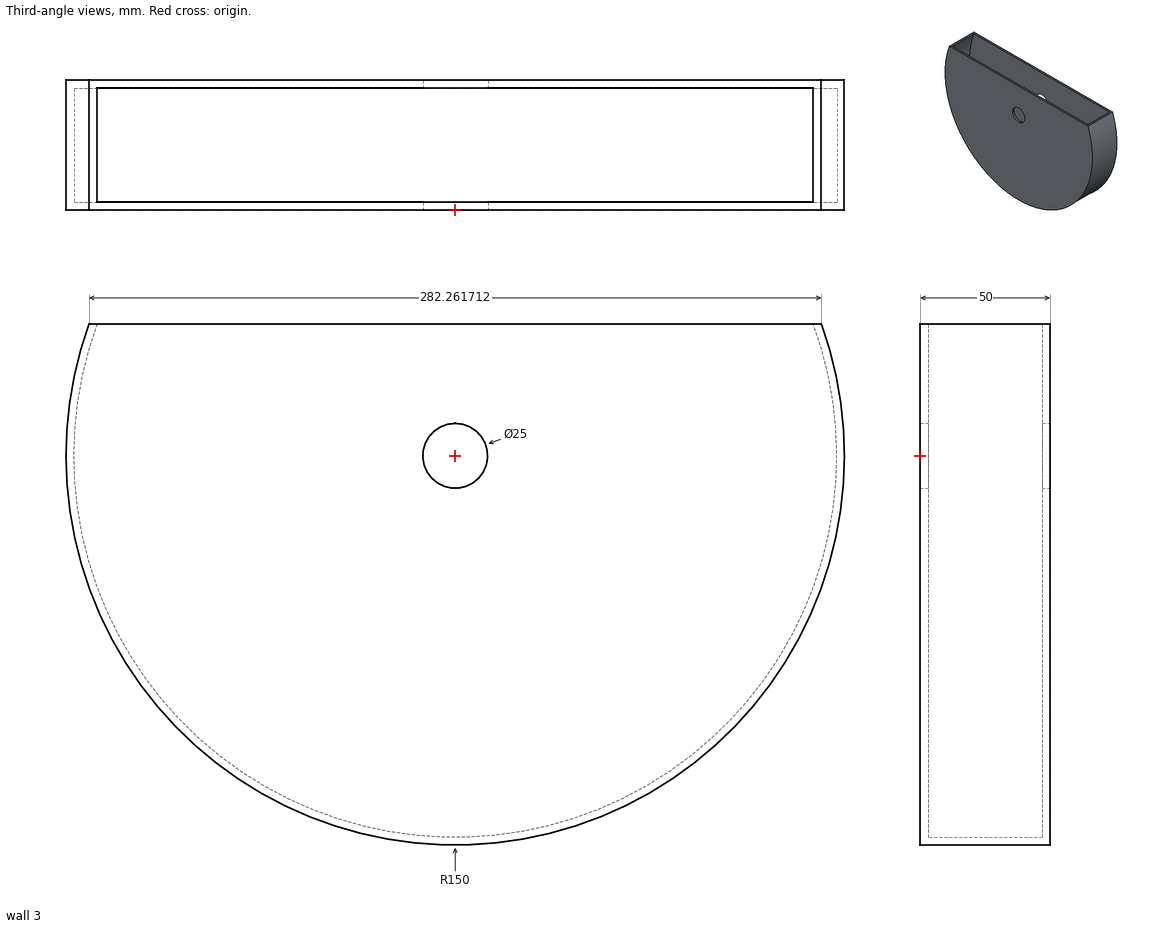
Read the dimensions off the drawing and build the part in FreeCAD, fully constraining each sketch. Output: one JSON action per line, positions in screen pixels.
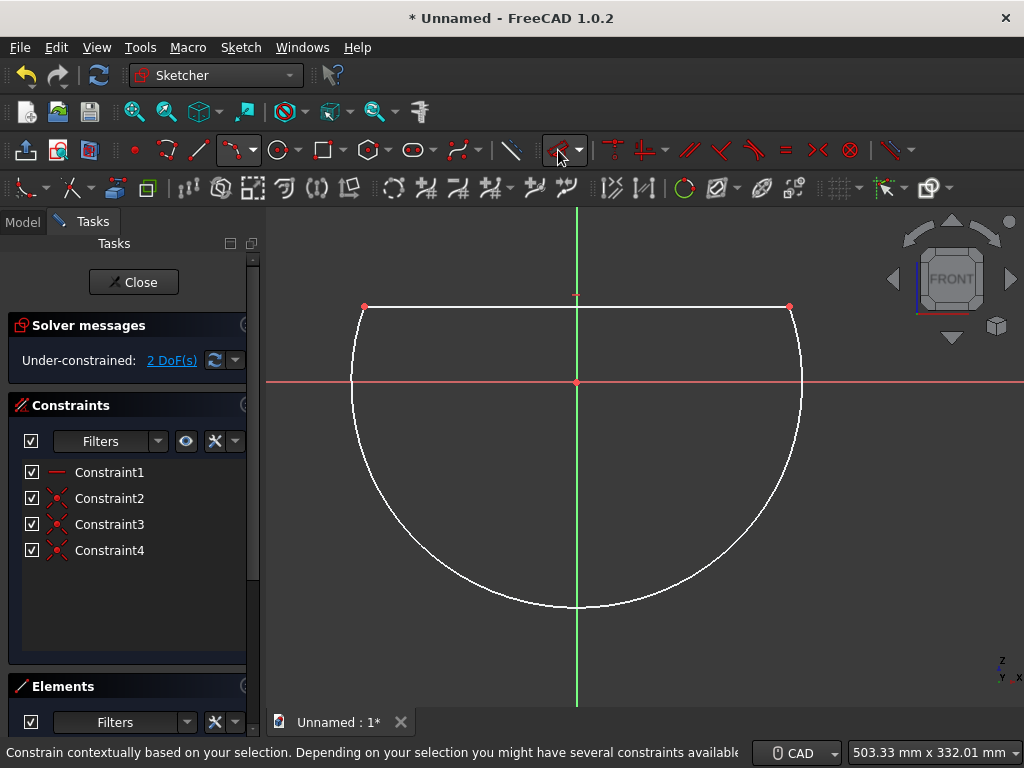
{"action": "left_click", "coordinate": [421, 545]}
{"action": "left_click", "coordinate": [399, 568]}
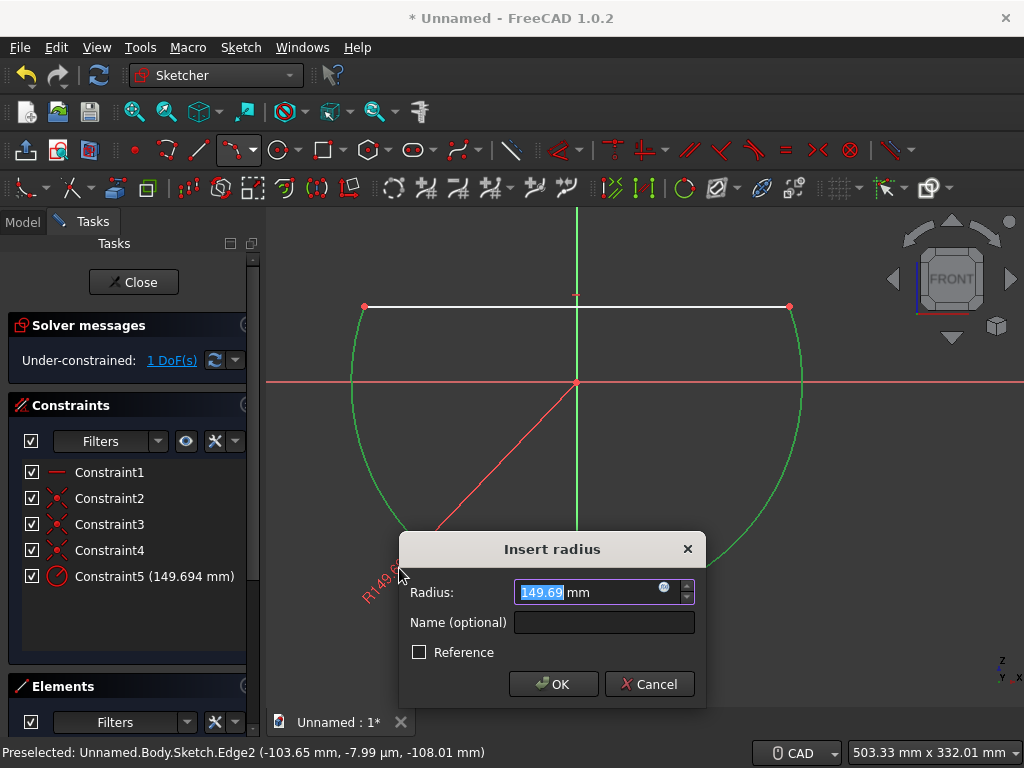
{"action": "type", "text": "150"}
{"action": "key", "text": "Return"}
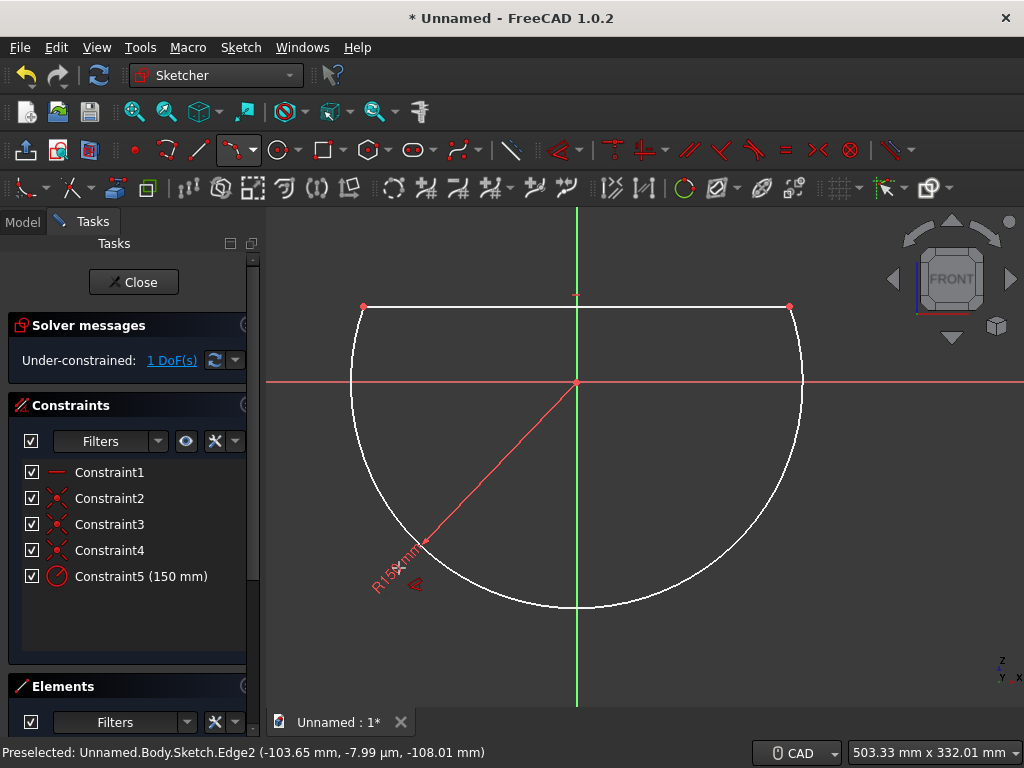
{"action": "left_click", "coordinate": [492, 307]}
{"action": "left_click", "coordinate": [479, 273]}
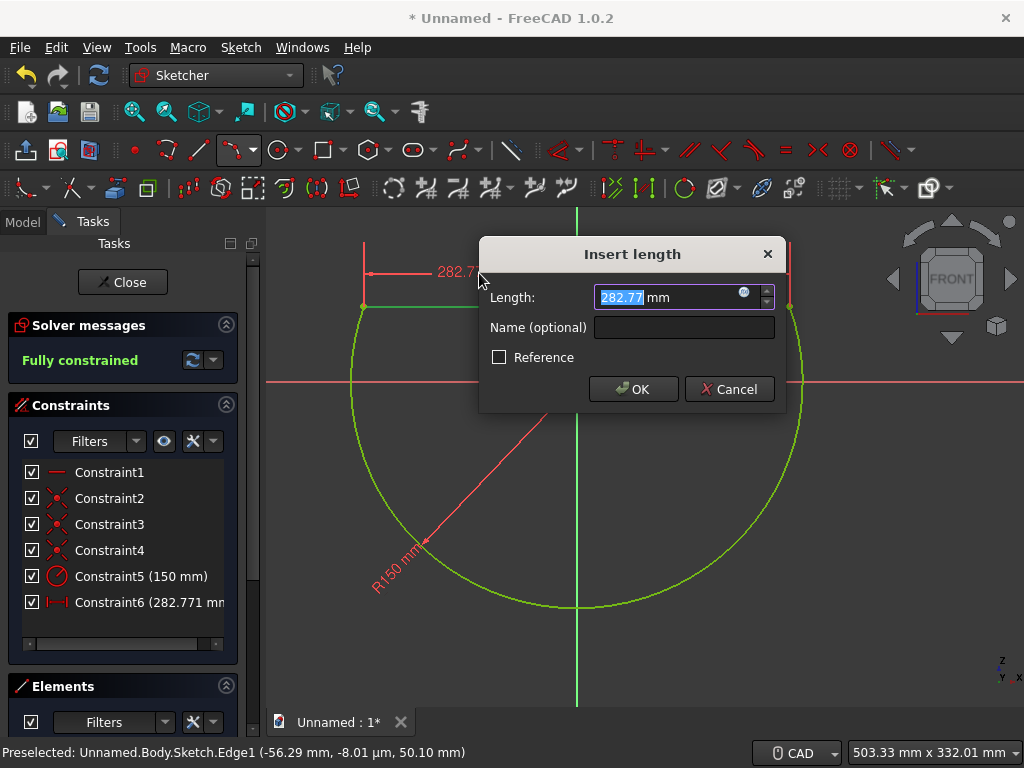
{"action": "type", "text": "282.261712"}
{"action": "key", "text": "Return"}
{"action": "key", "text": "Escape"}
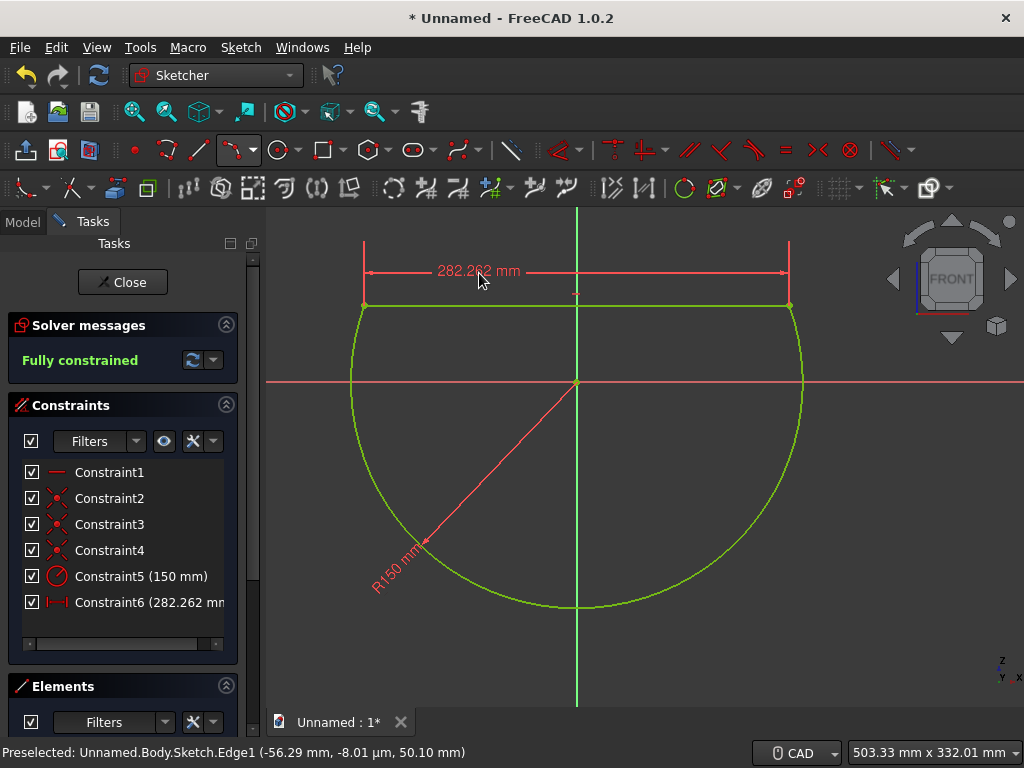
{"action": "left_click", "coordinate": [123, 282]}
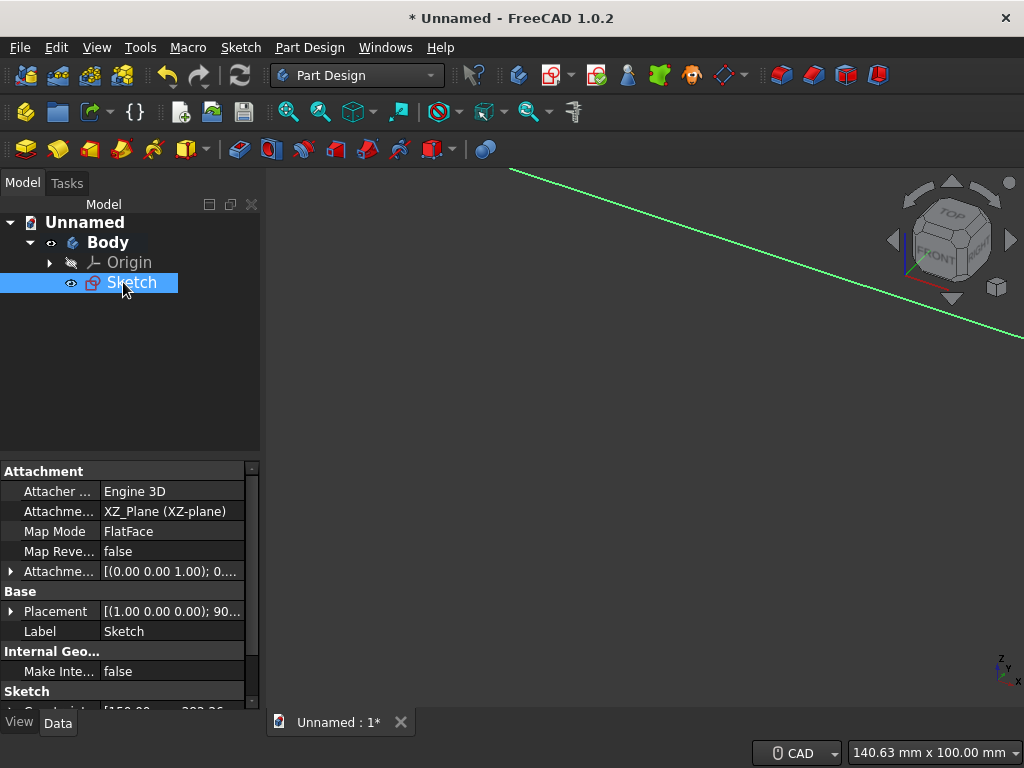
{"action": "left_click", "coordinate": [26, 150]}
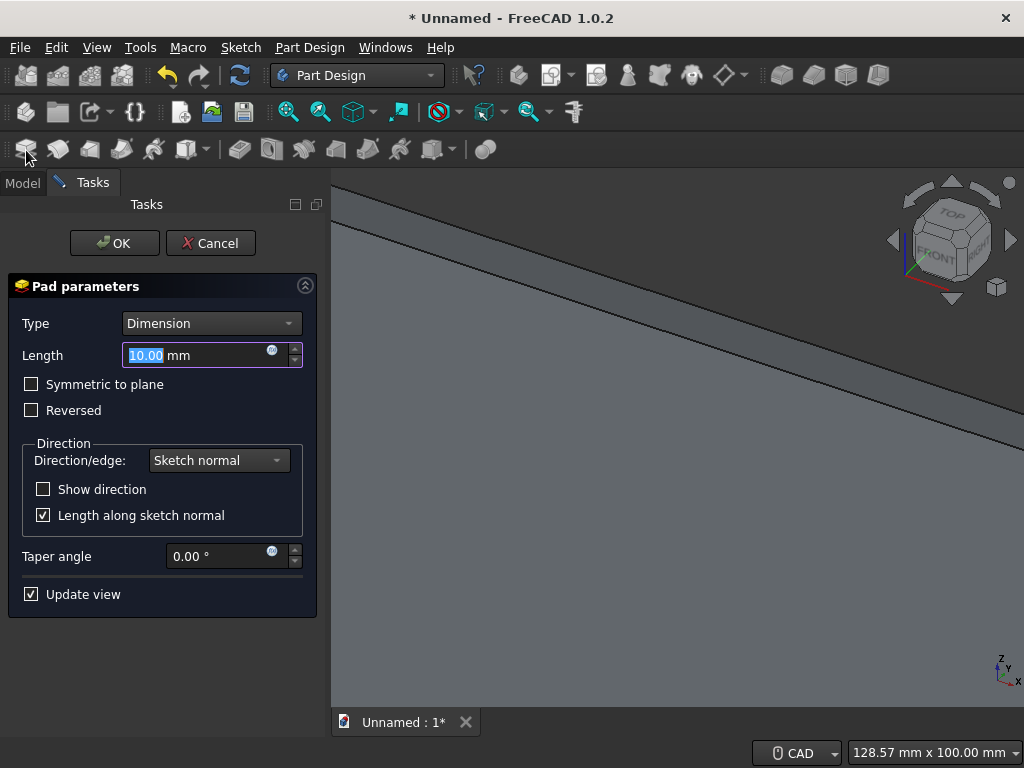
{"action": "type", "text": "50"}
{"action": "key", "text": "Tab"}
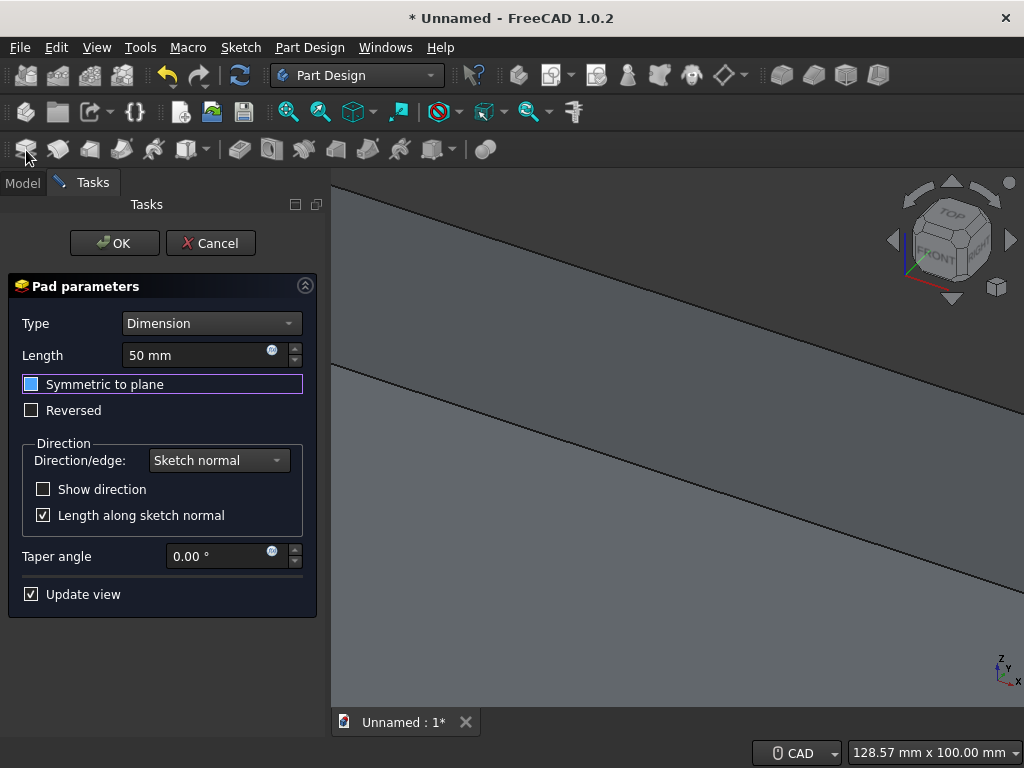
{"action": "left_click", "coordinate": [30, 410]}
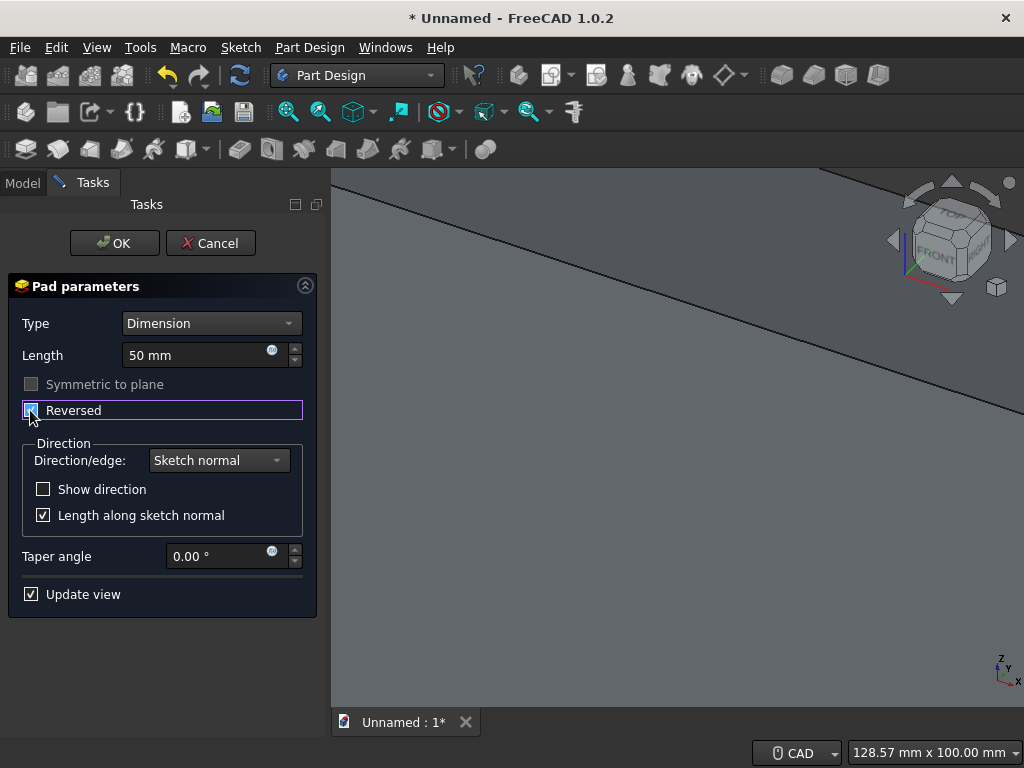
{"action": "left_click", "coordinate": [115, 243]}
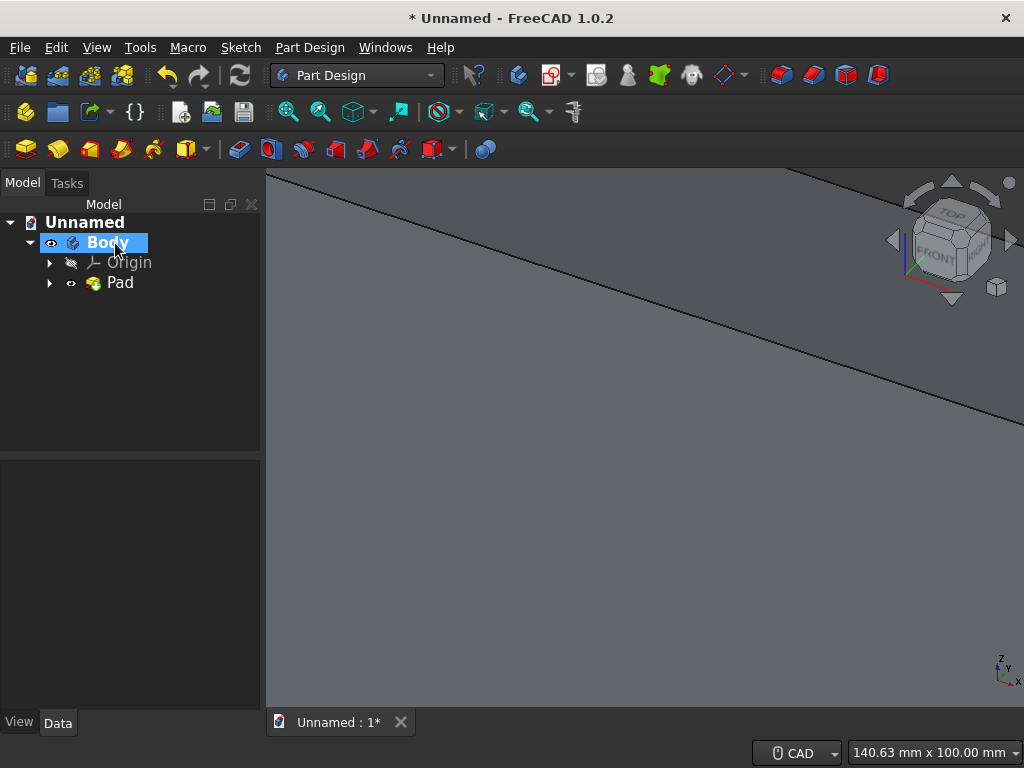
{"action": "left_click", "coordinate": [290, 112]}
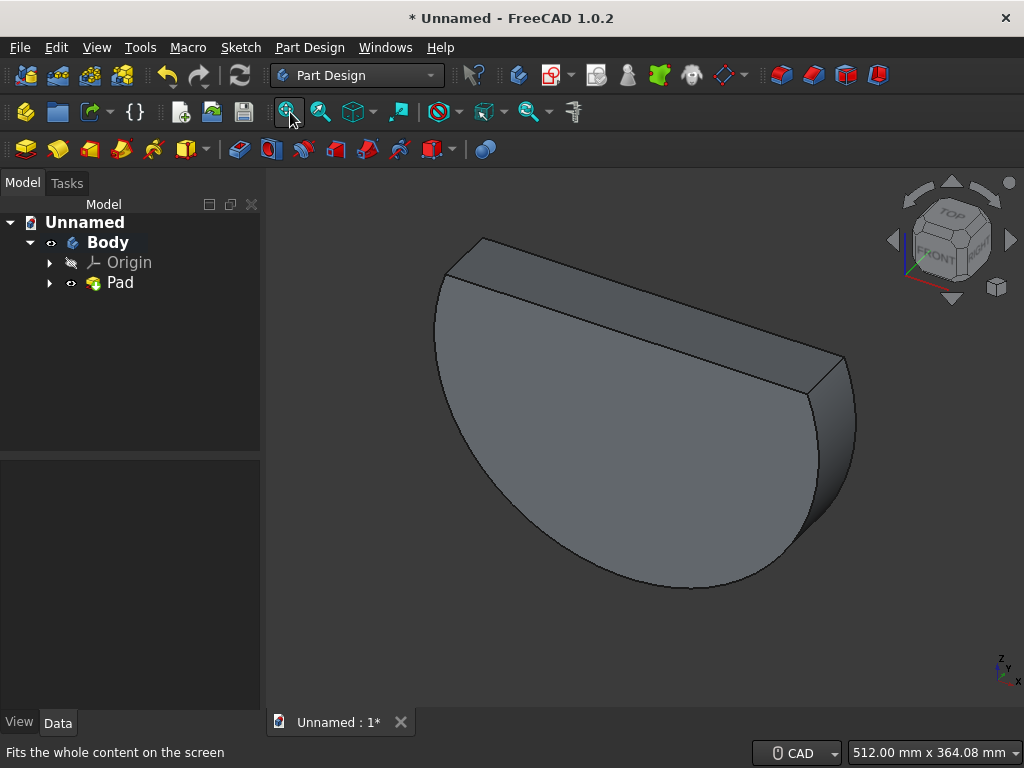
{"action": "left_click", "coordinate": [748, 349]}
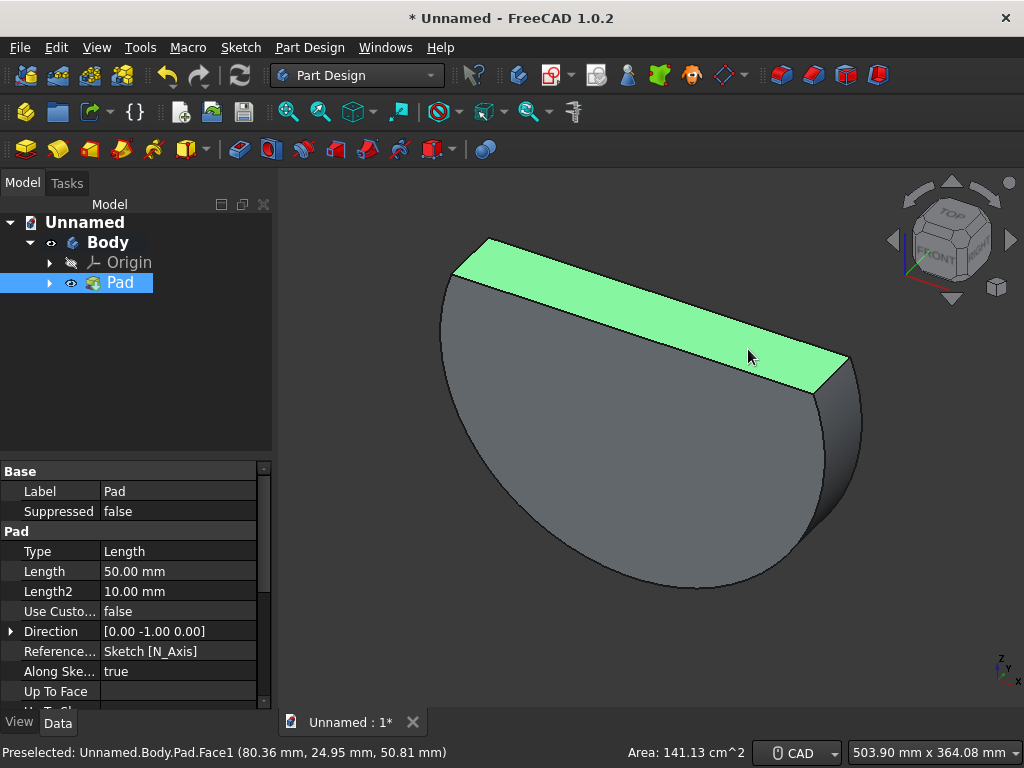
{"action": "left_click", "coordinate": [878, 76]}